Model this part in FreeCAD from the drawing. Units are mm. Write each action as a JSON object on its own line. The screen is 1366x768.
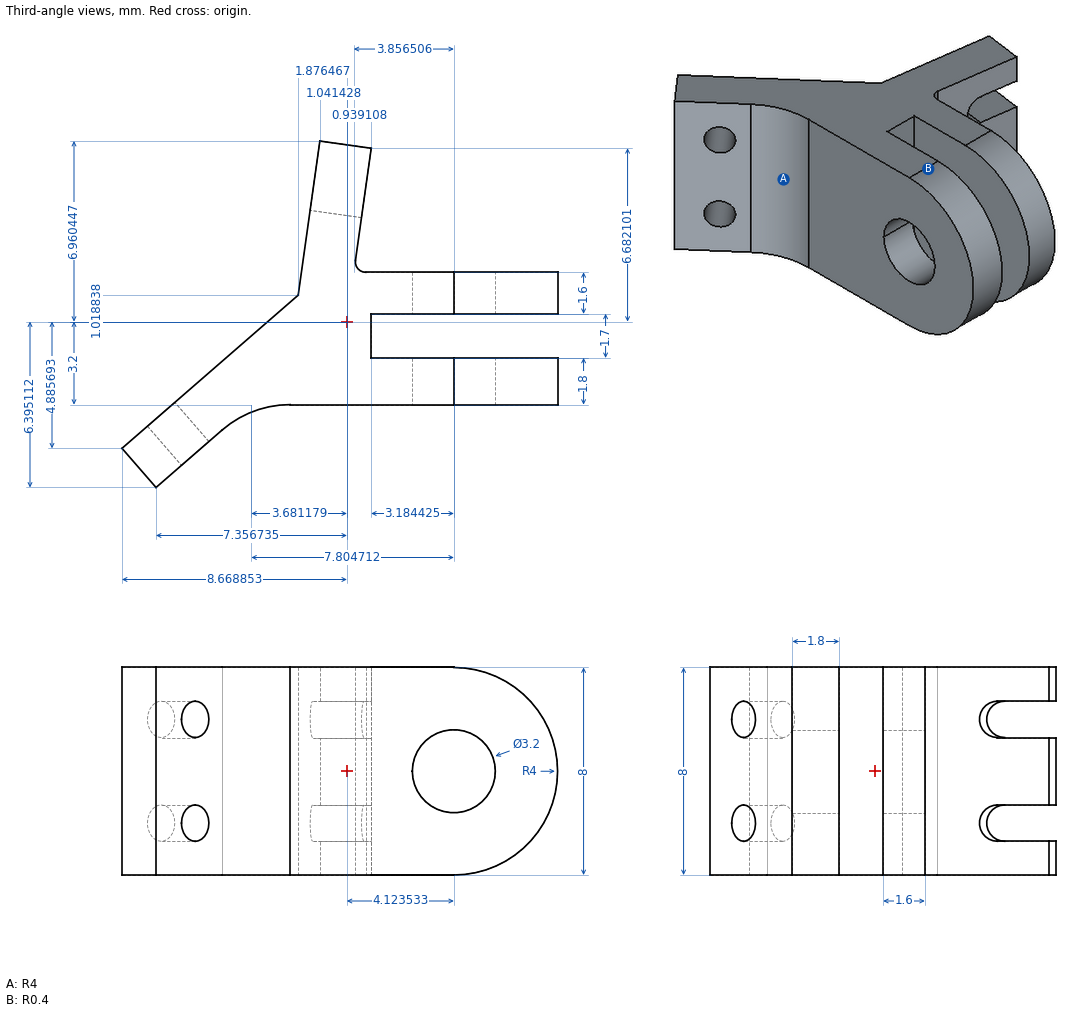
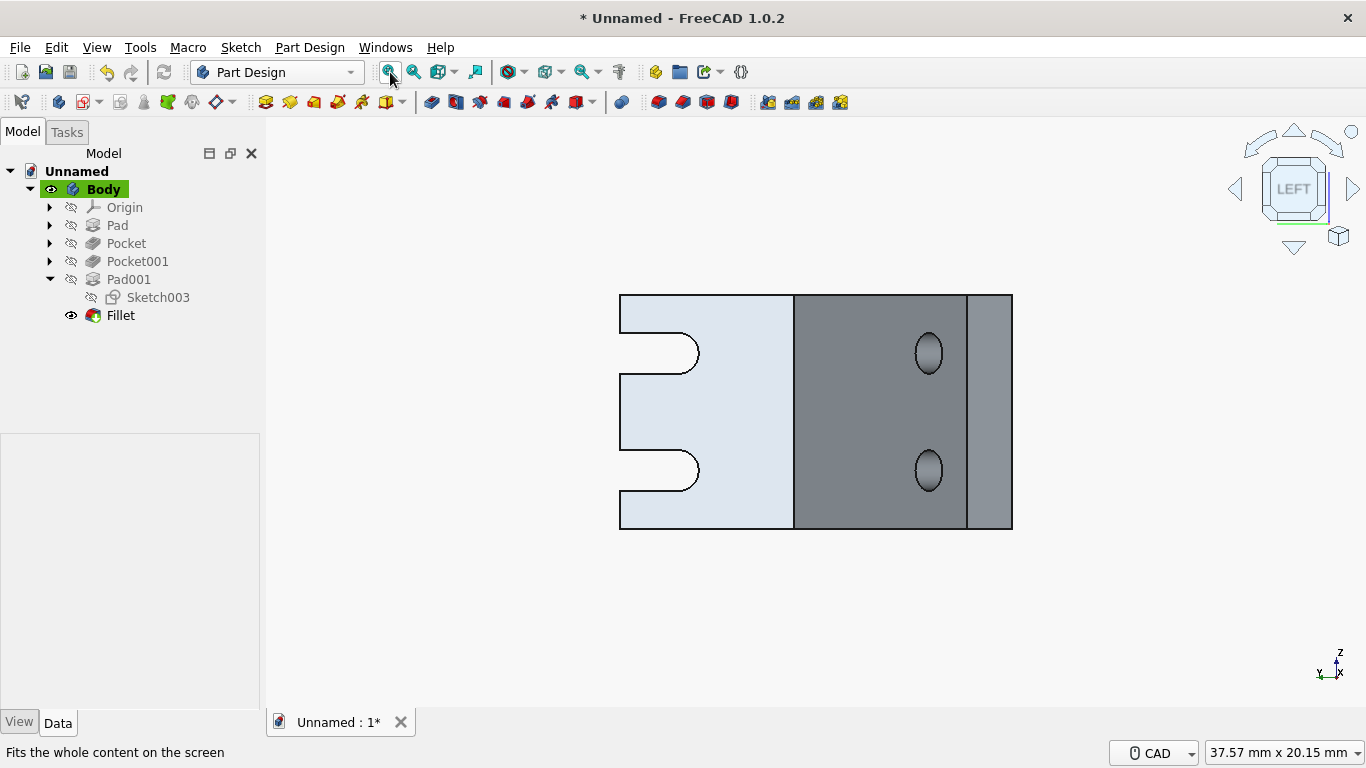
{"action": "key", "text": "v 3"}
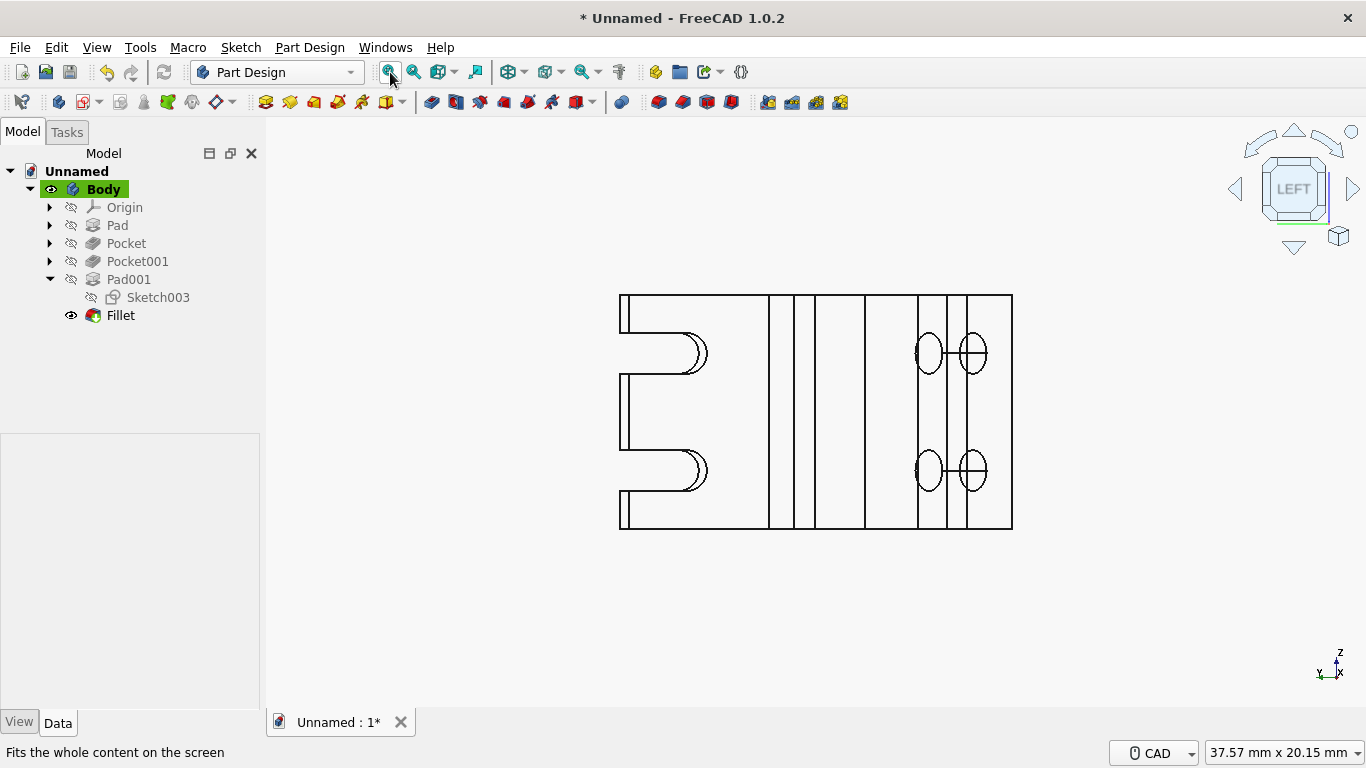
{"action": "key", "text": "0"}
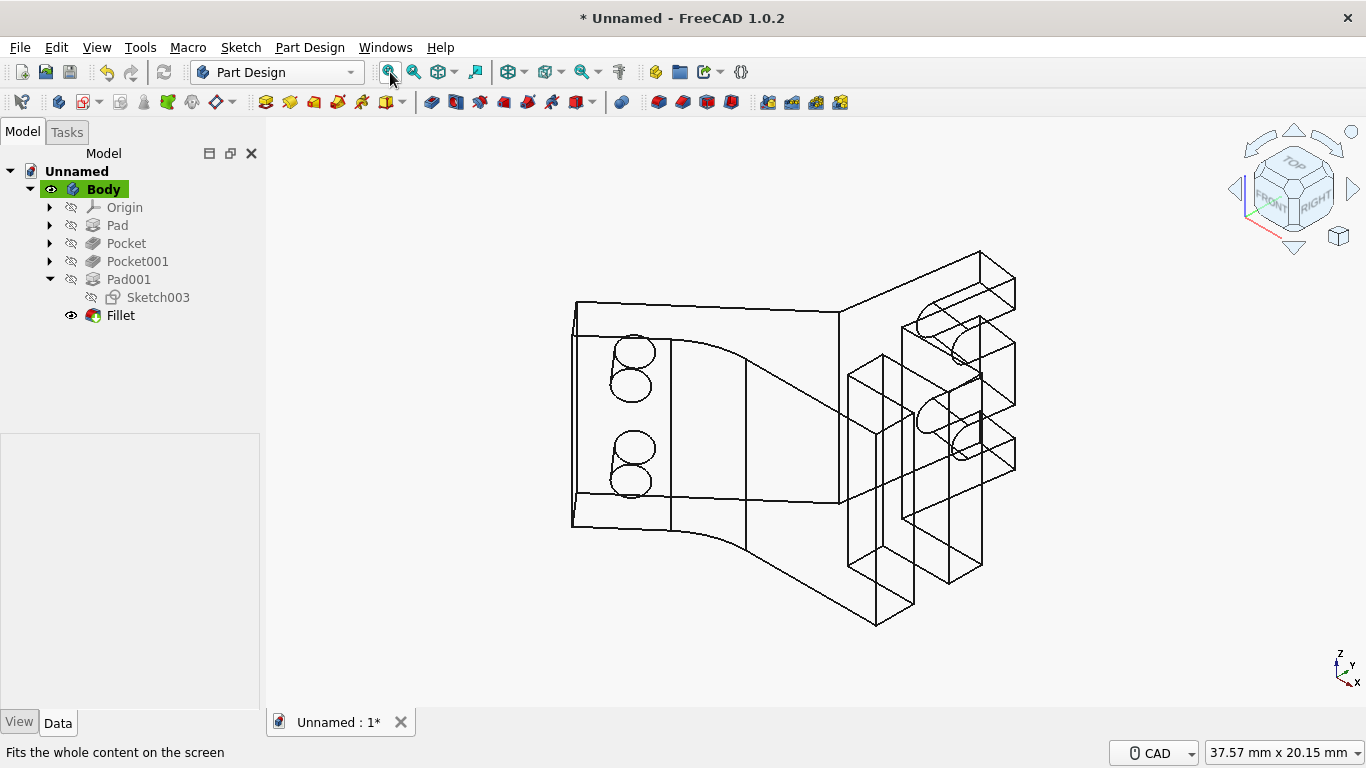
{"action": "left_click", "coordinate": [902, 441]}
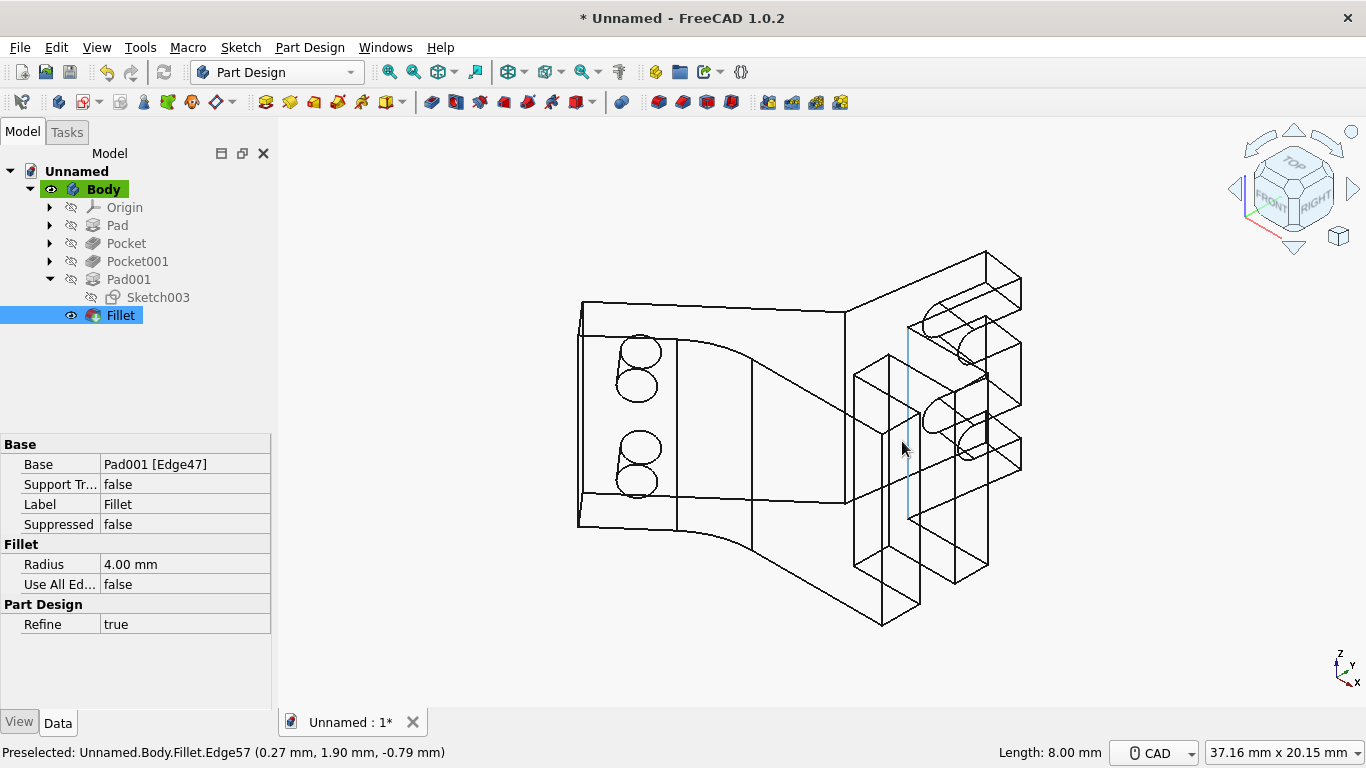
{"action": "key", "text": "v 1"}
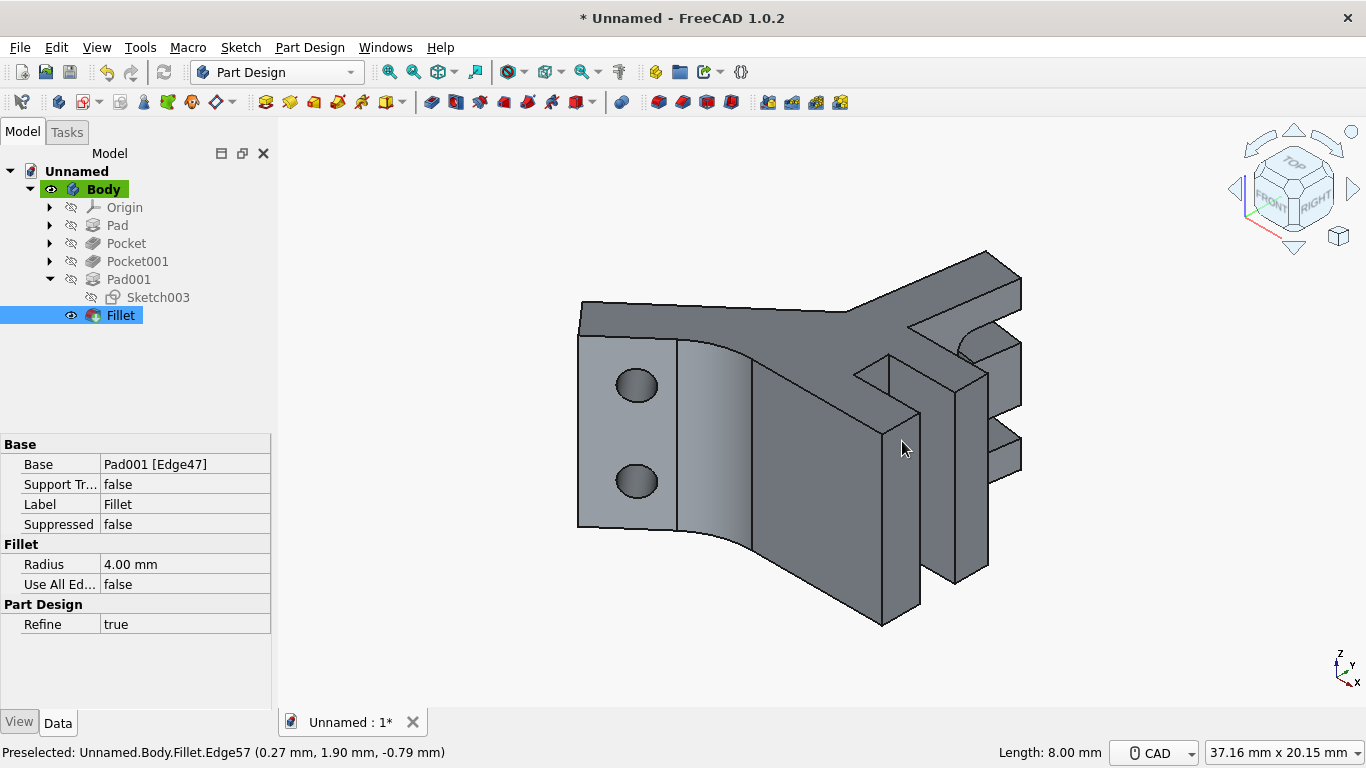
{"action": "left_click", "coordinate": [660, 102]}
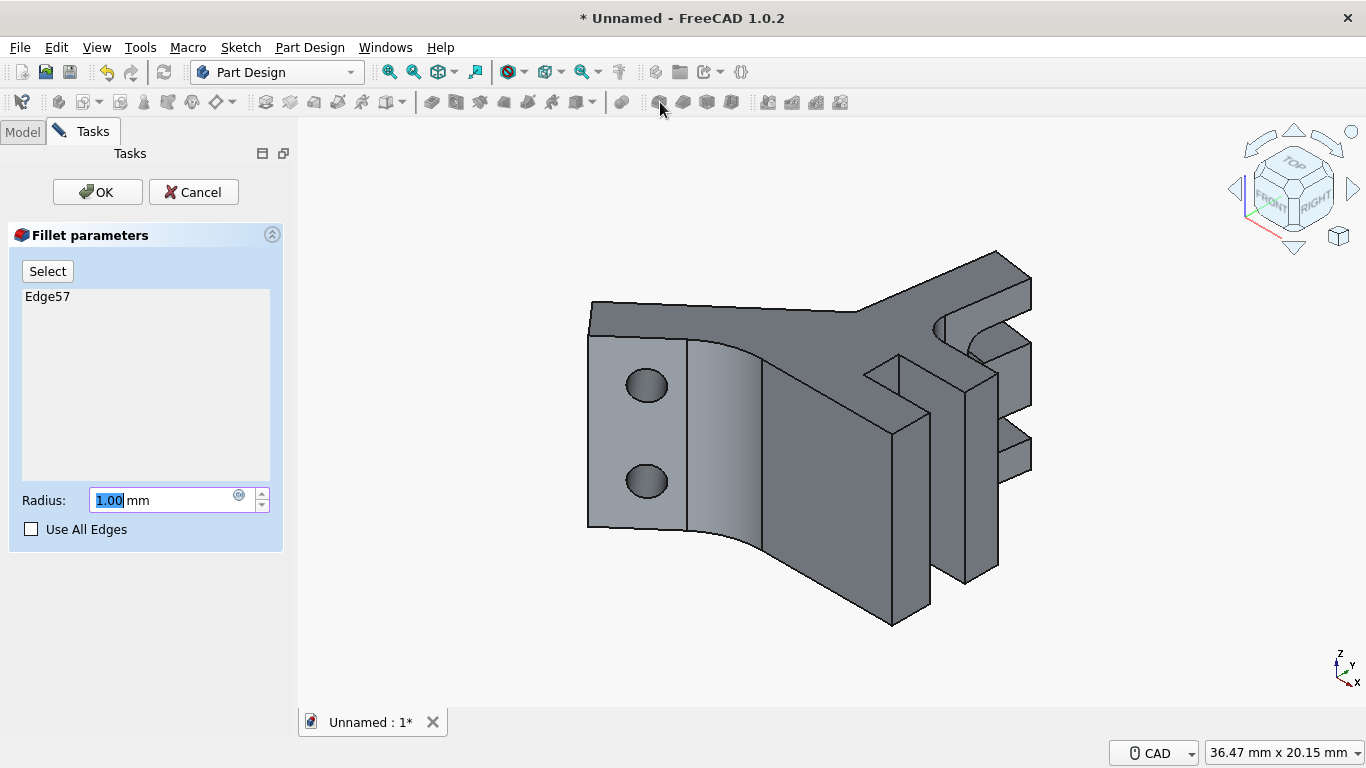
{"action": "type", "text": "0.4"}
{"action": "key", "text": "Tab"}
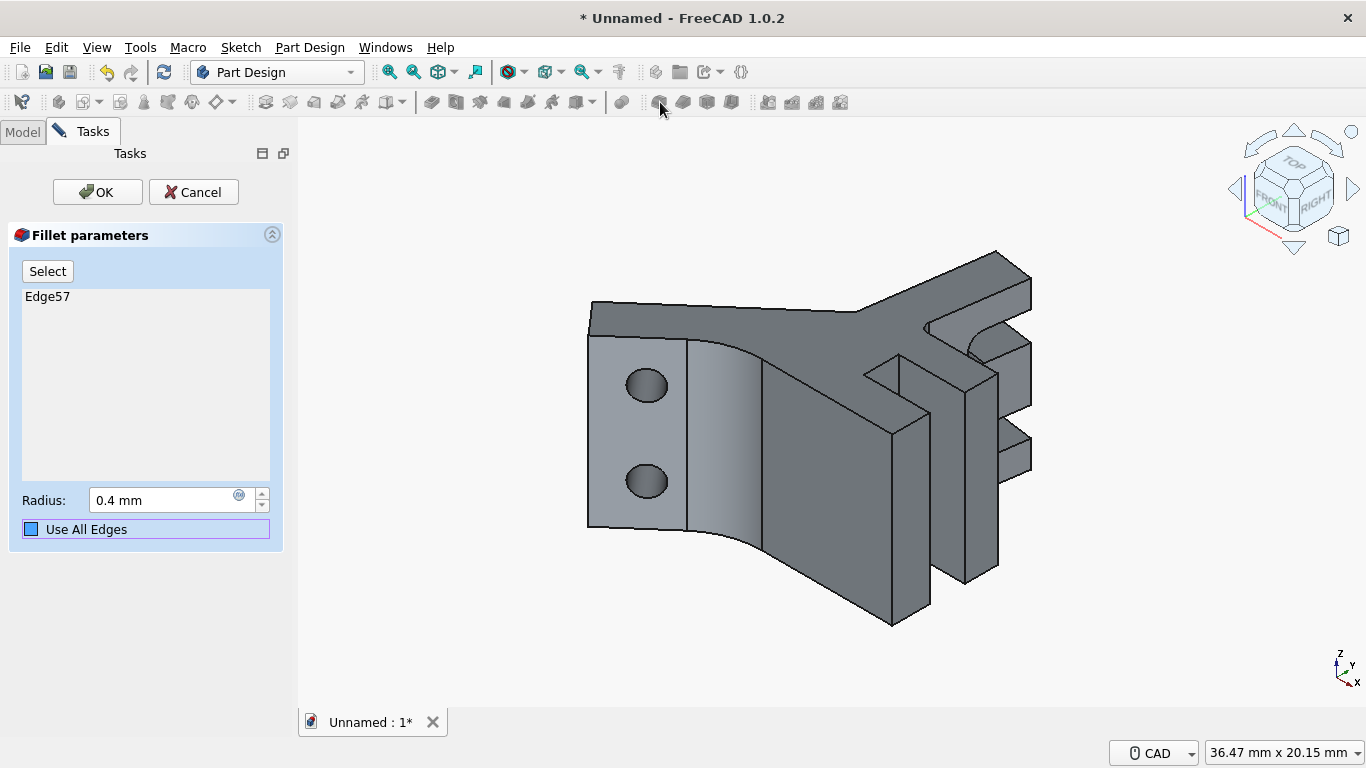
{"action": "left_click", "coordinate": [98, 192]}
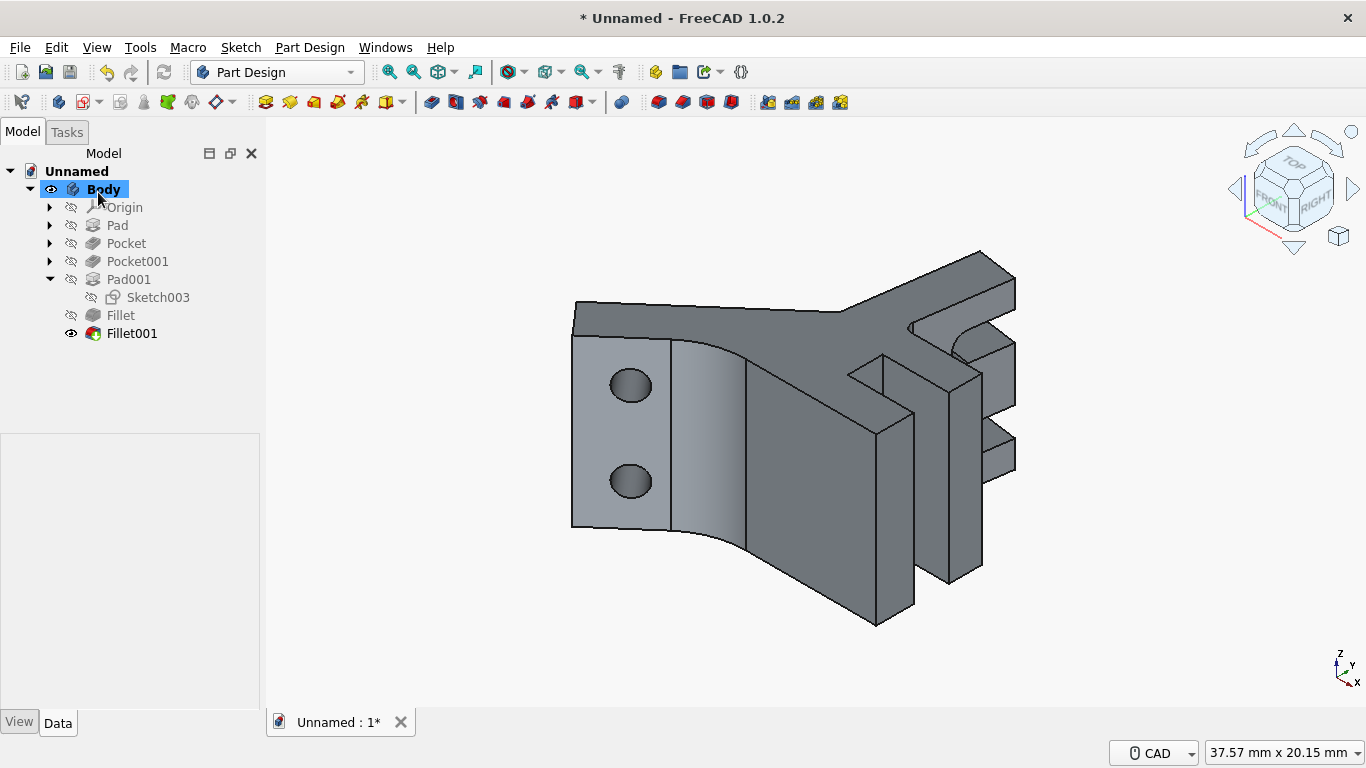
{"action": "left_click", "coordinate": [50, 207]}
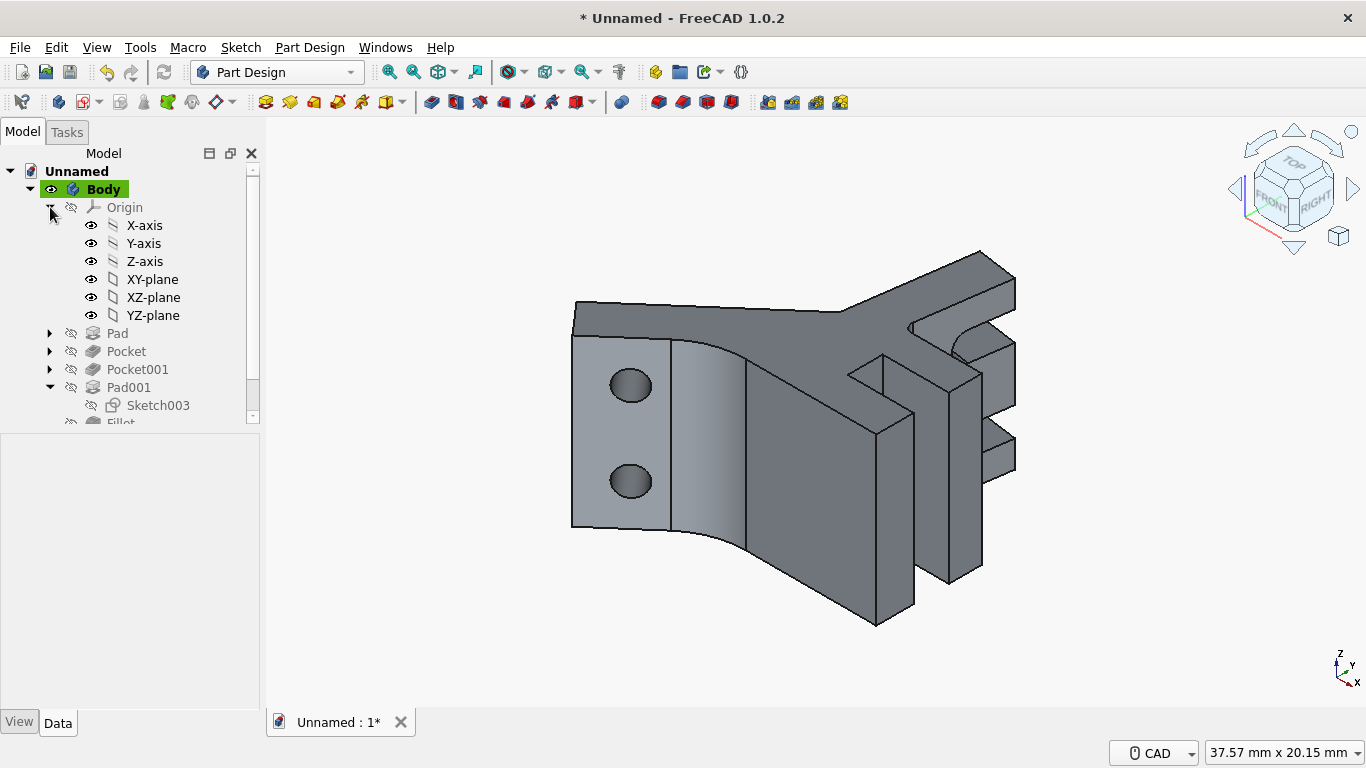
{"action": "left_click", "coordinate": [136, 297]}